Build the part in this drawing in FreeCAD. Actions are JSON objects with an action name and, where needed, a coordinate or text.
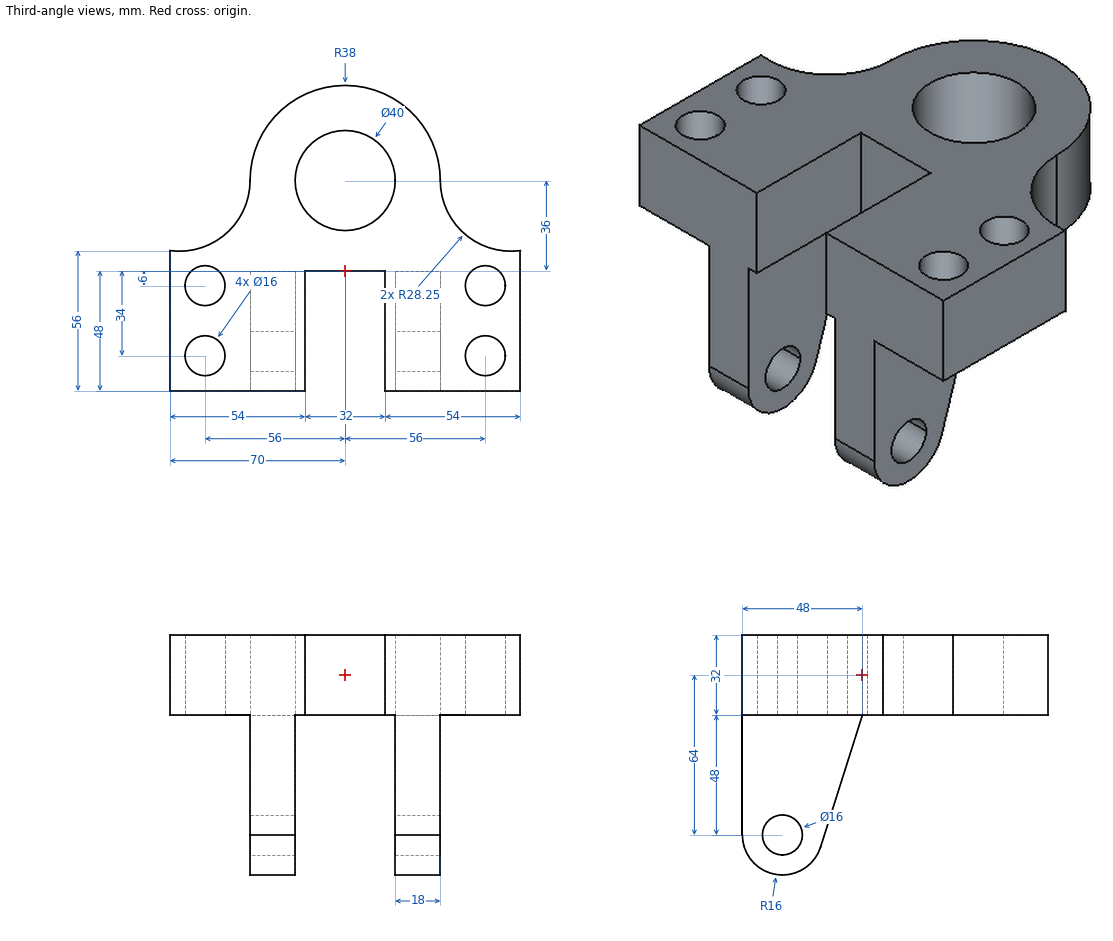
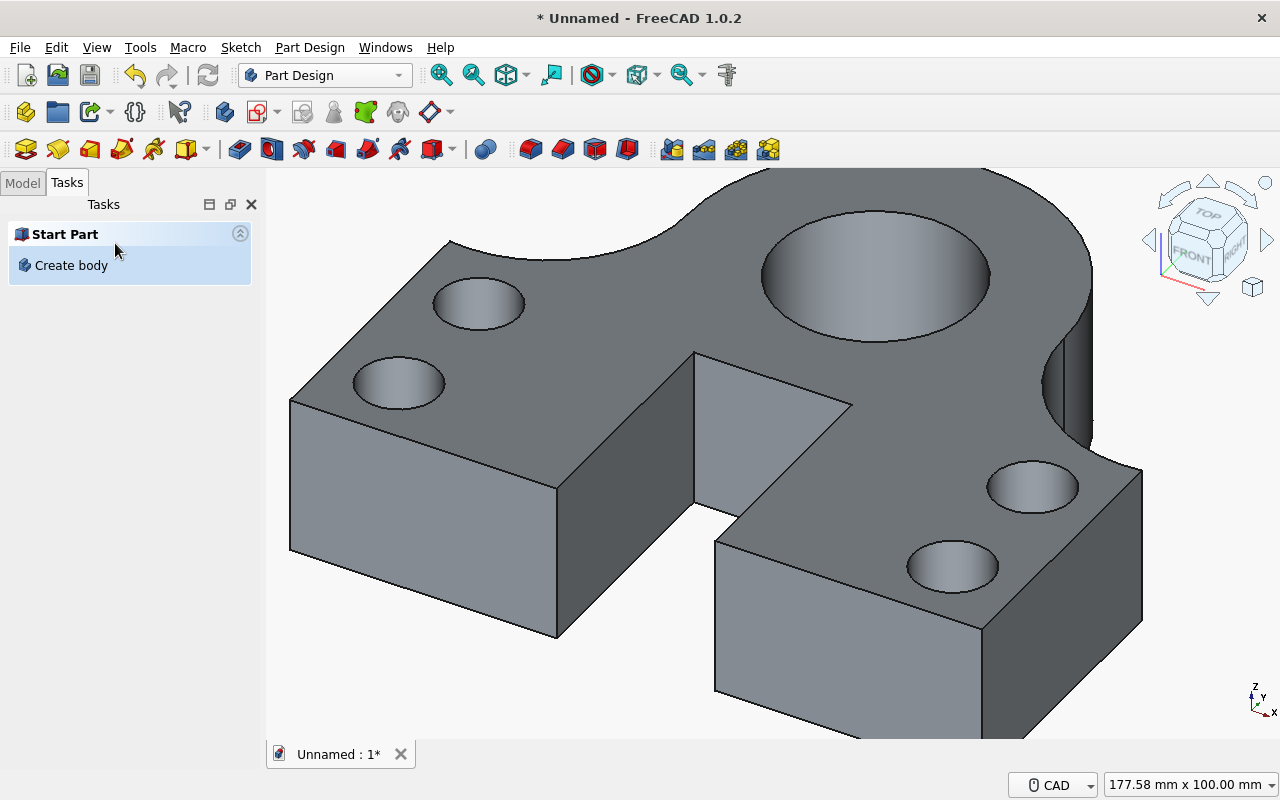
{"action": "left_click", "coordinate": [442, 76]}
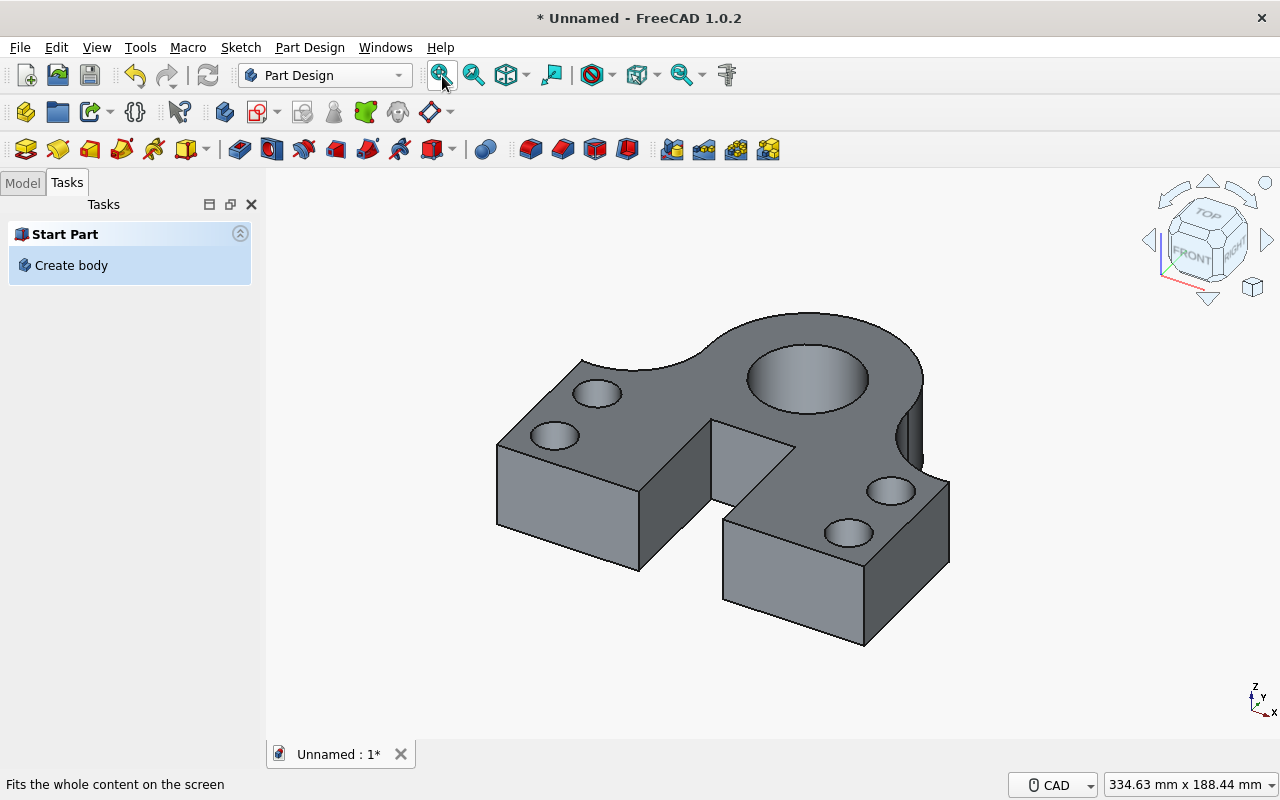
{"action": "left_click", "coordinate": [23, 182]}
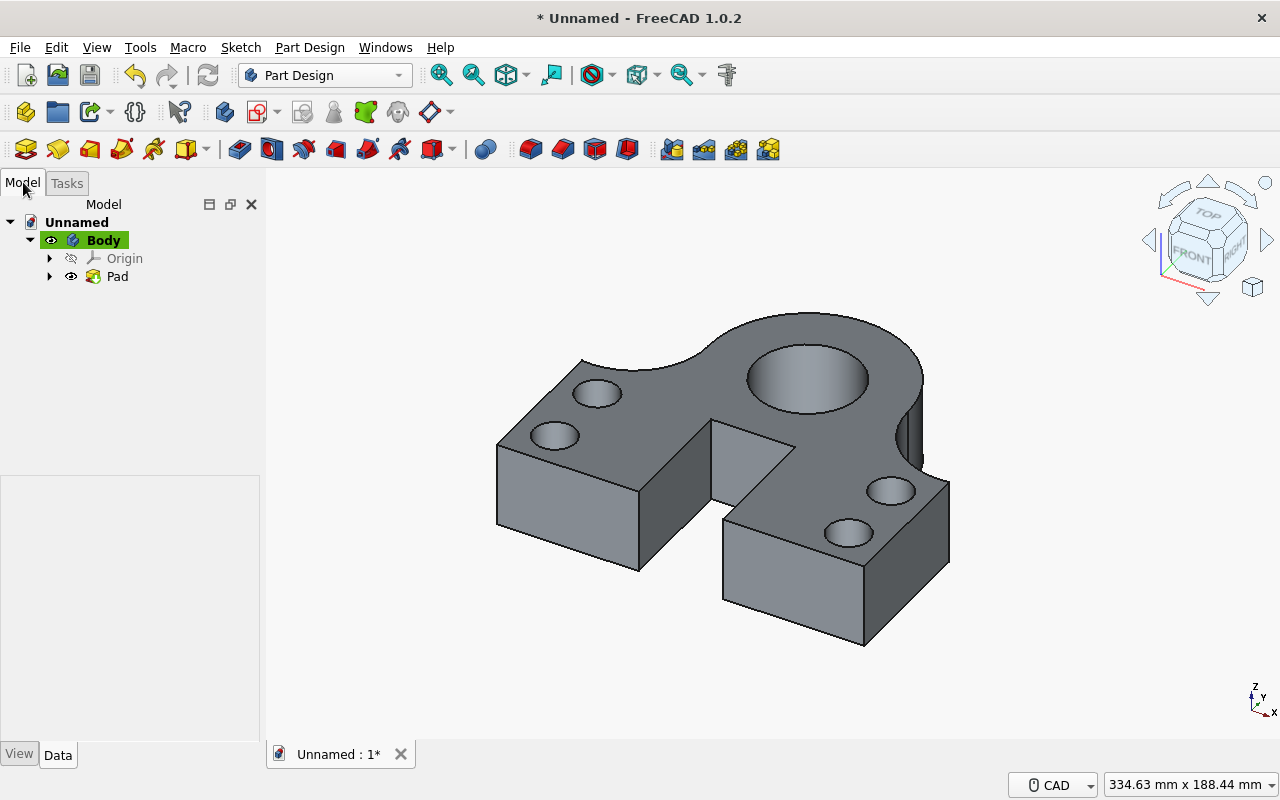
{"action": "left_click", "coordinate": [50, 258]}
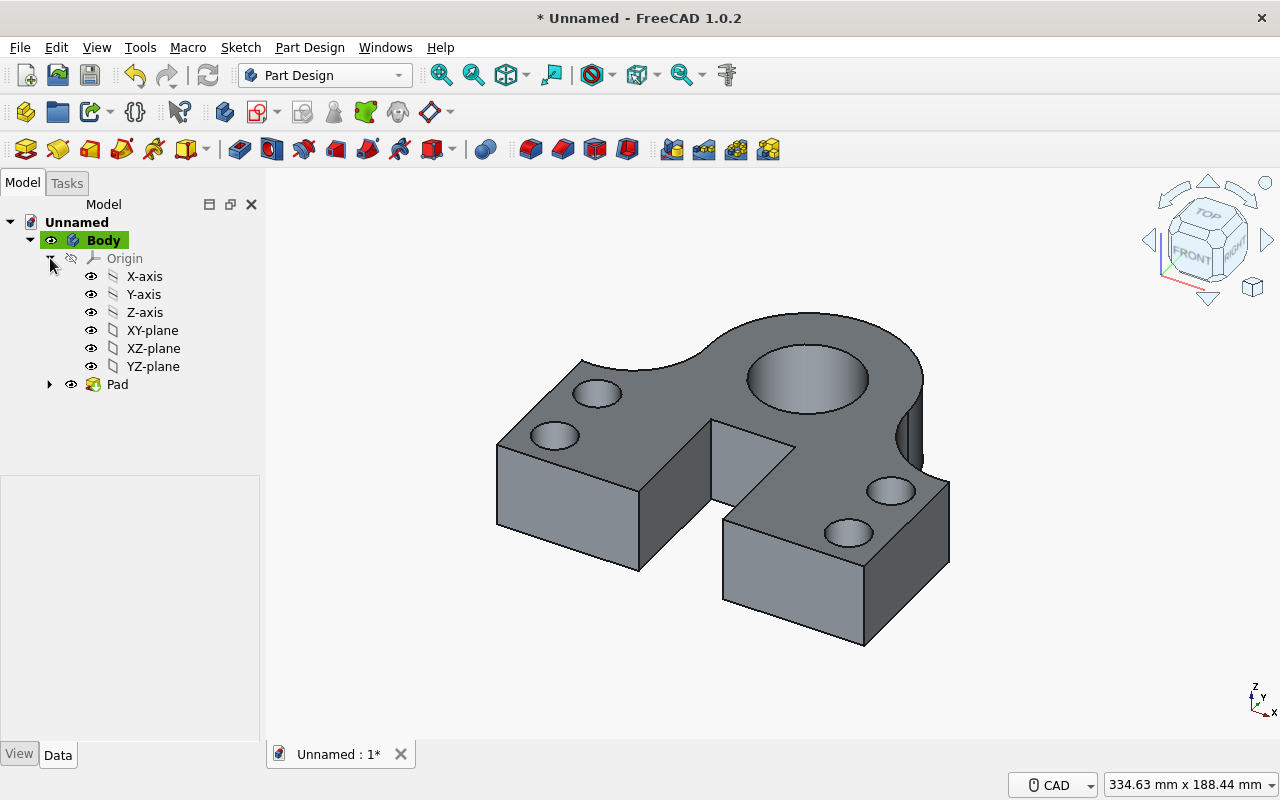
{"action": "left_click", "coordinate": [136, 366]}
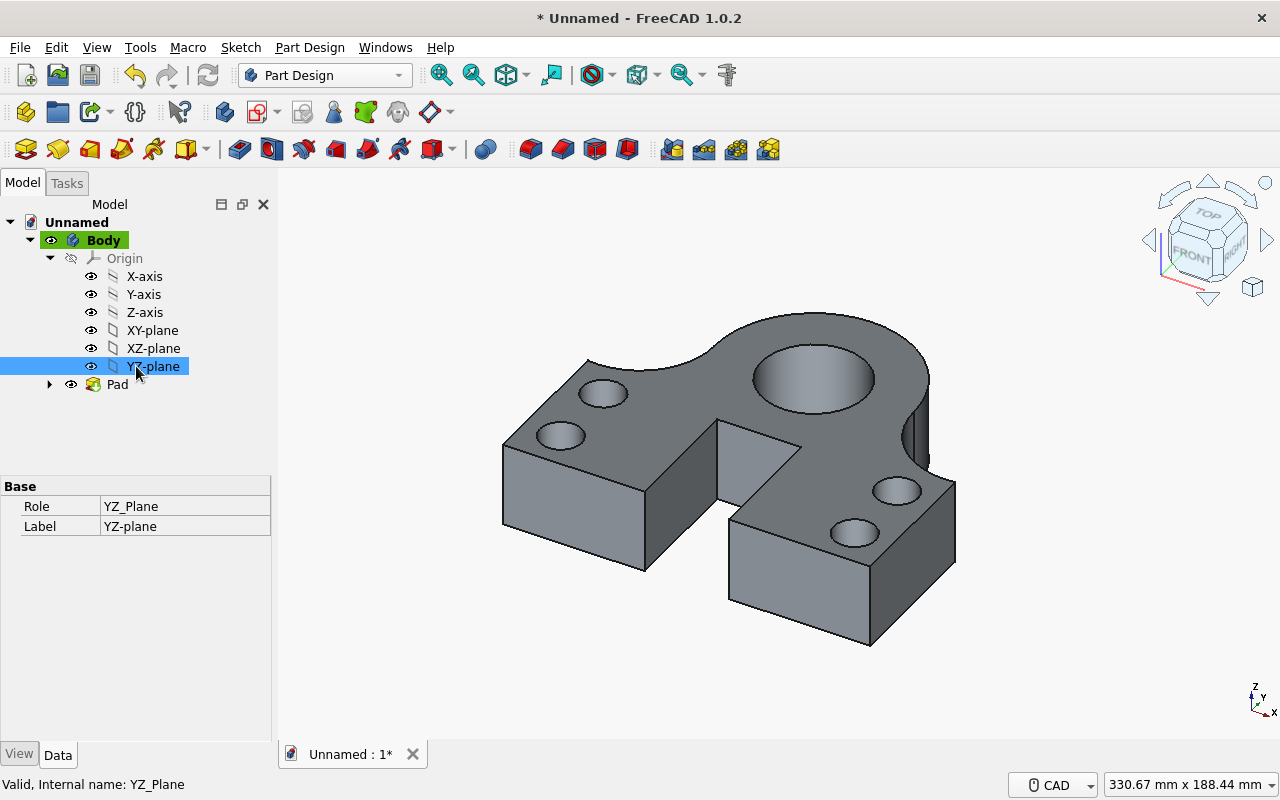
{"action": "left_click", "coordinate": [430, 112]}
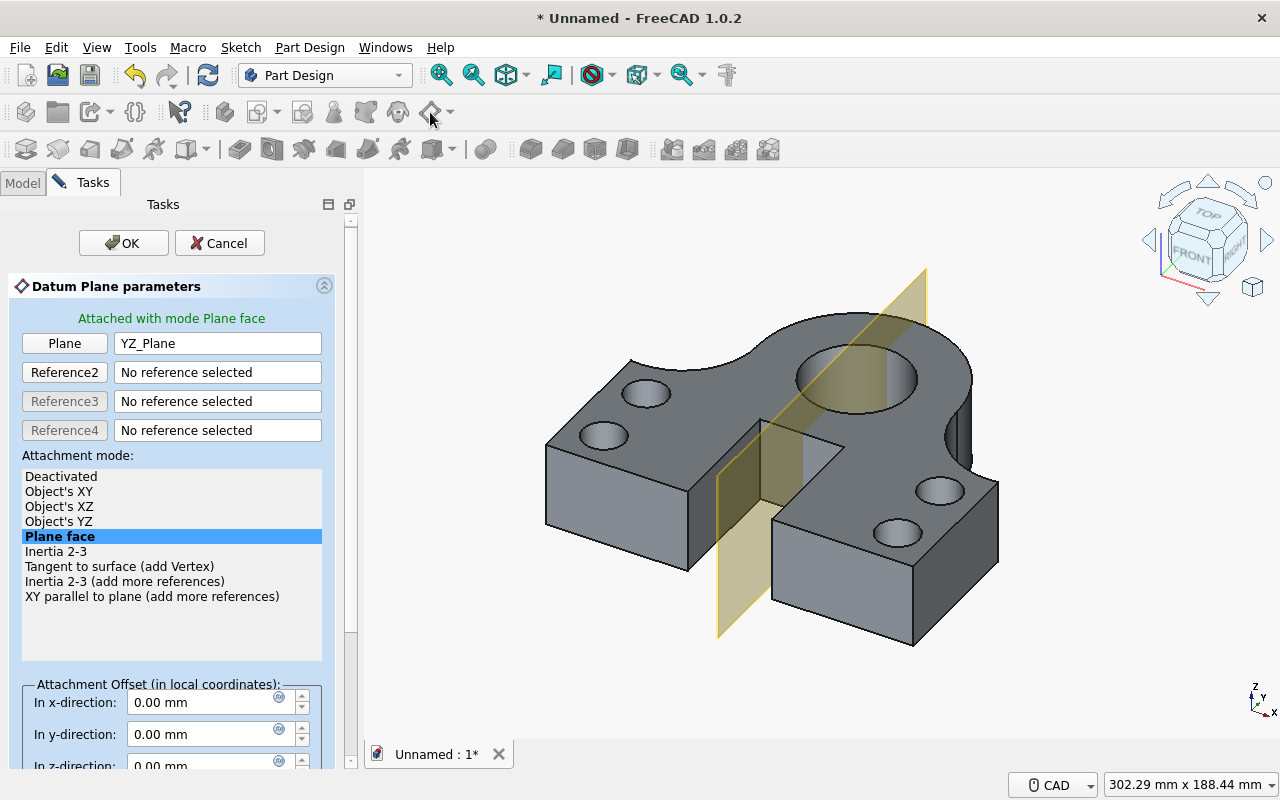
{"action": "scroll", "coordinate": [351, 491], "scroll_direction": "down", "scroll_amount": 2}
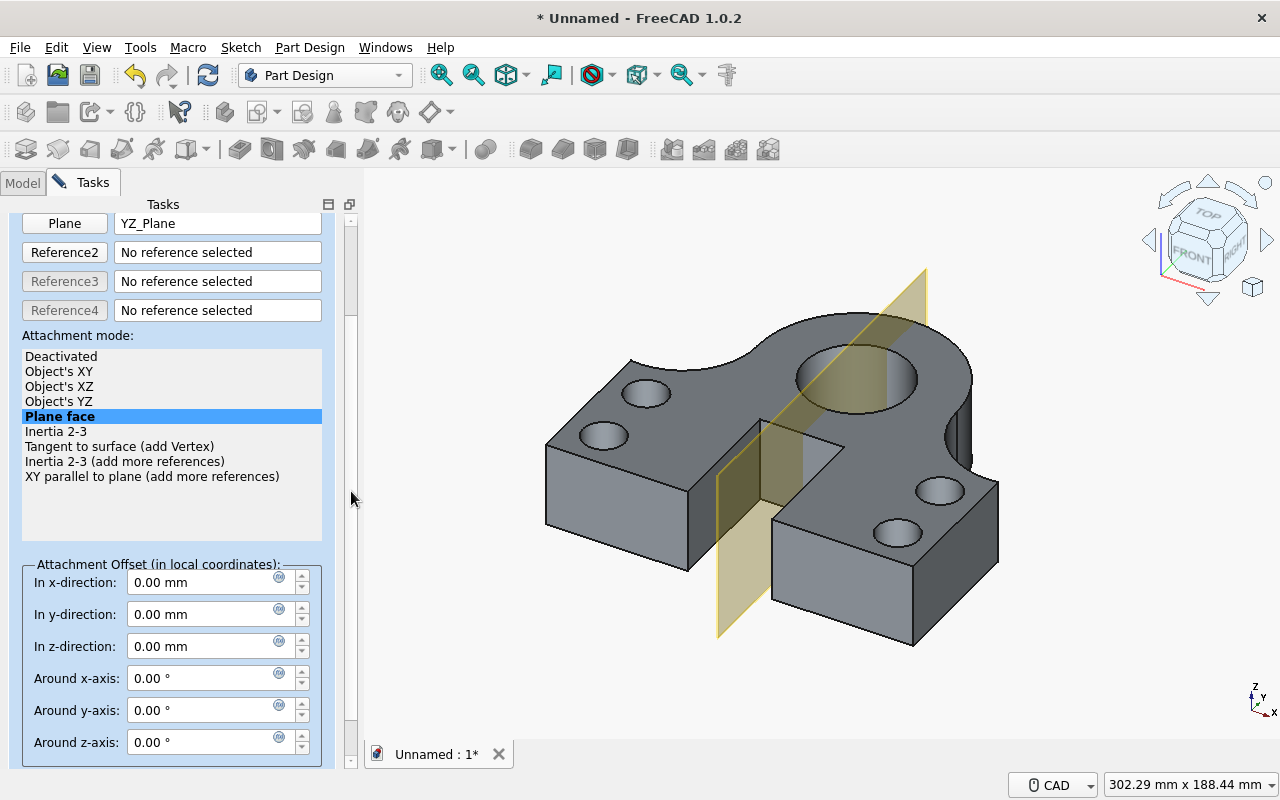
{"action": "triple_click", "coordinate": [210, 646]}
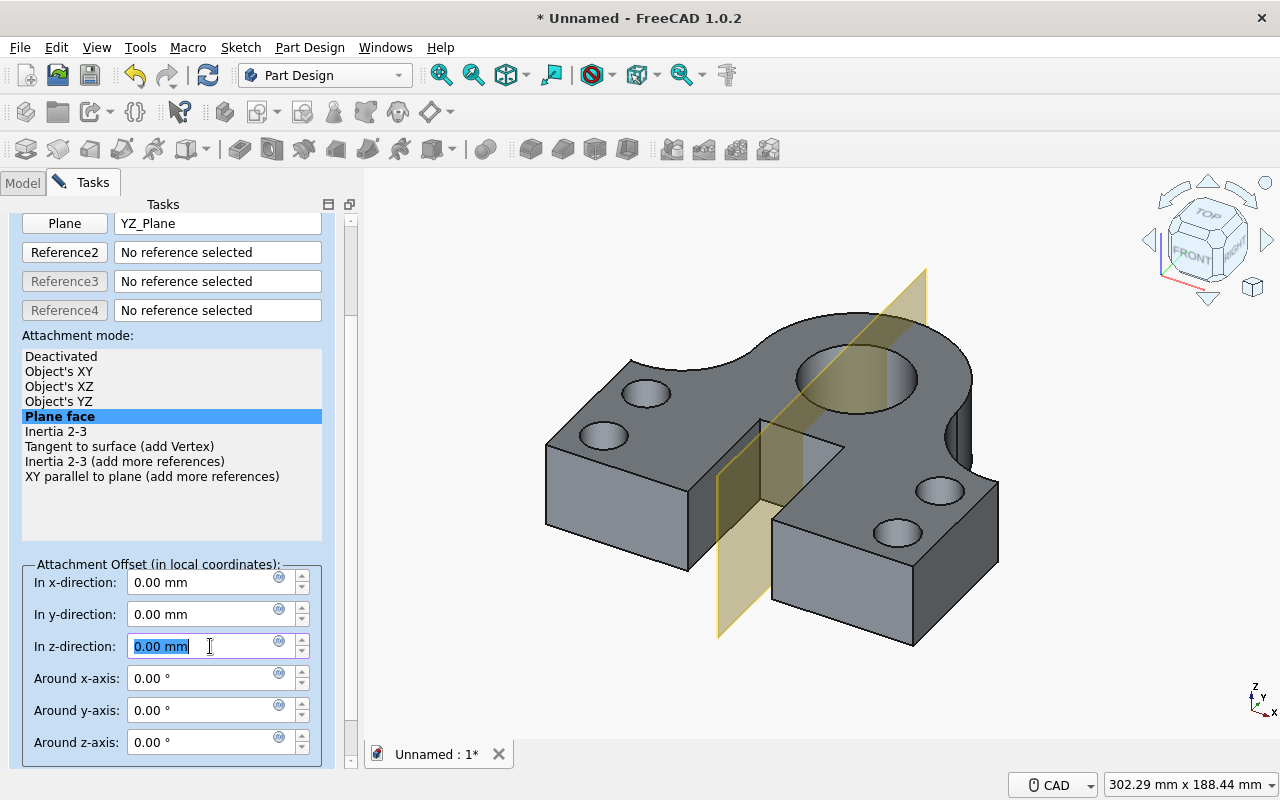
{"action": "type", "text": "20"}
{"action": "key", "text": "Tab"}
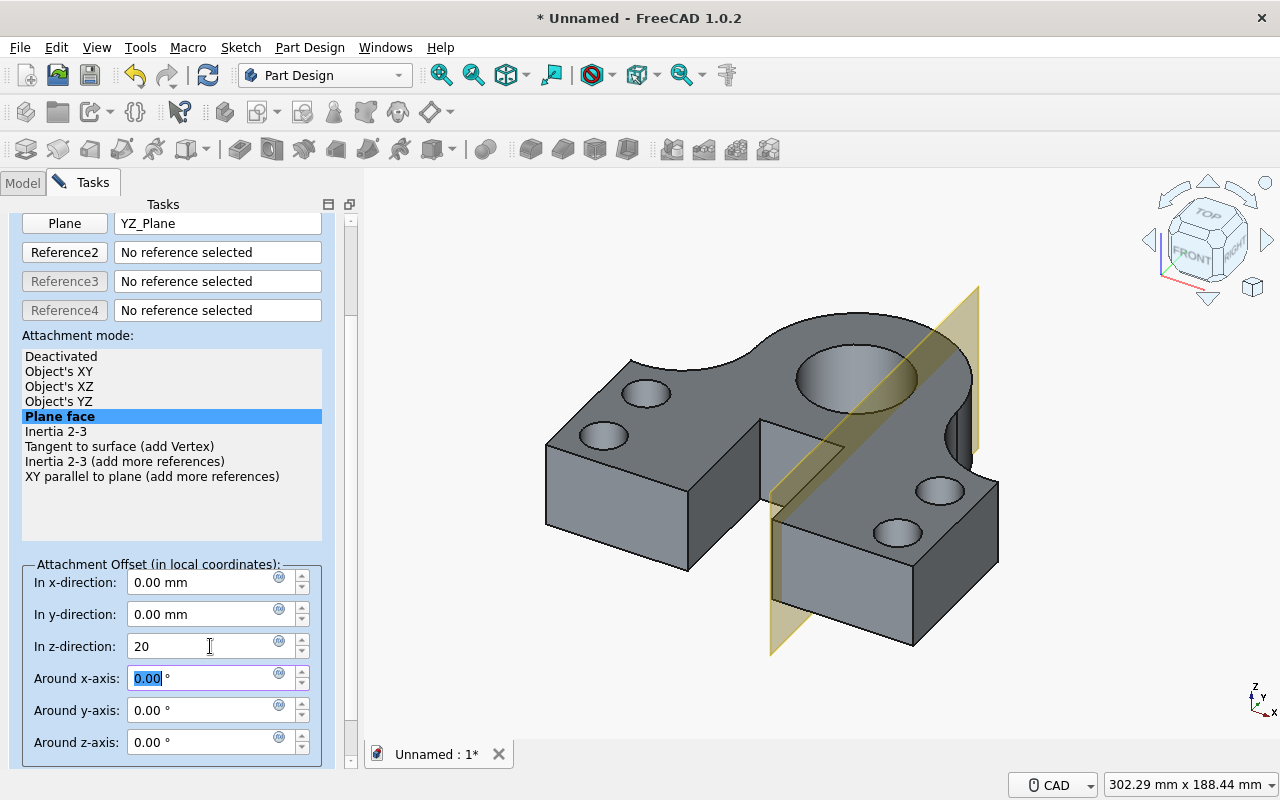
{"action": "scroll", "coordinate": [351, 491], "scroll_direction": "up", "scroll_amount": 3}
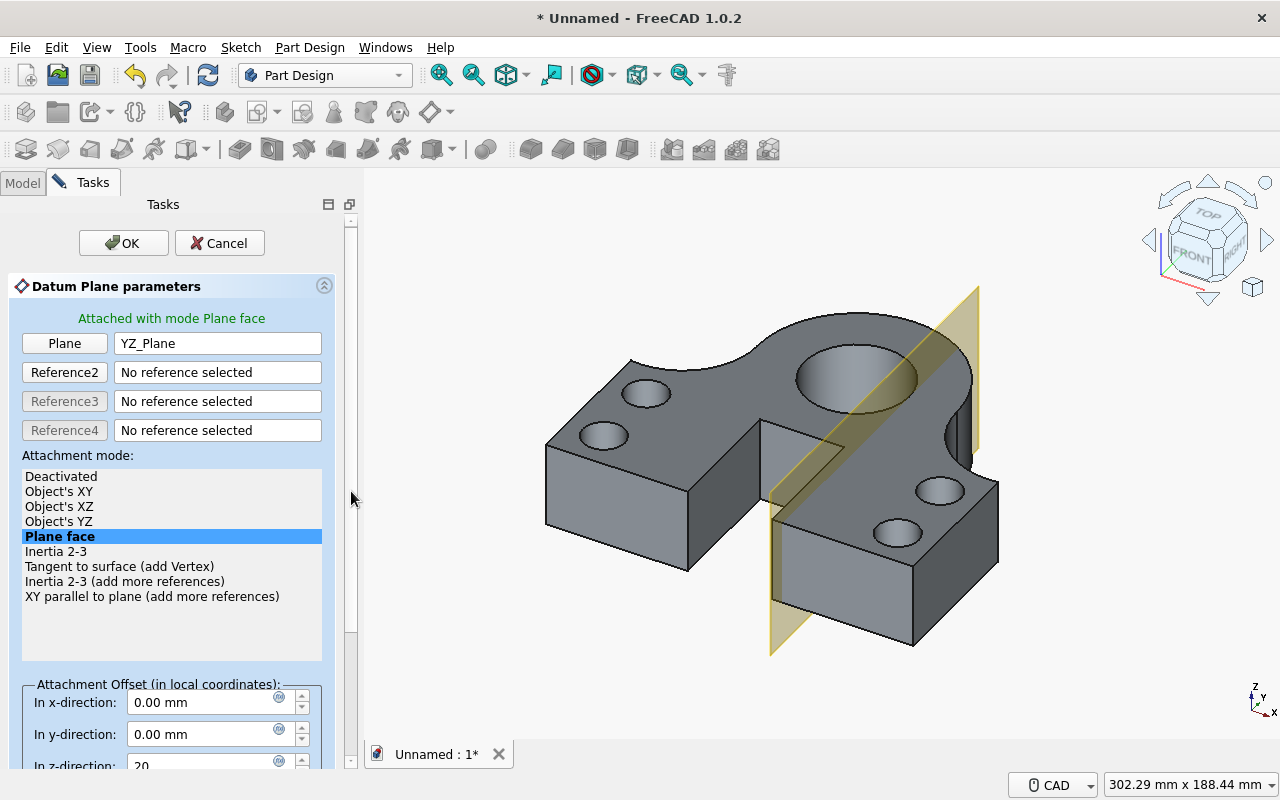
{"action": "left_click", "coordinate": [124, 243]}